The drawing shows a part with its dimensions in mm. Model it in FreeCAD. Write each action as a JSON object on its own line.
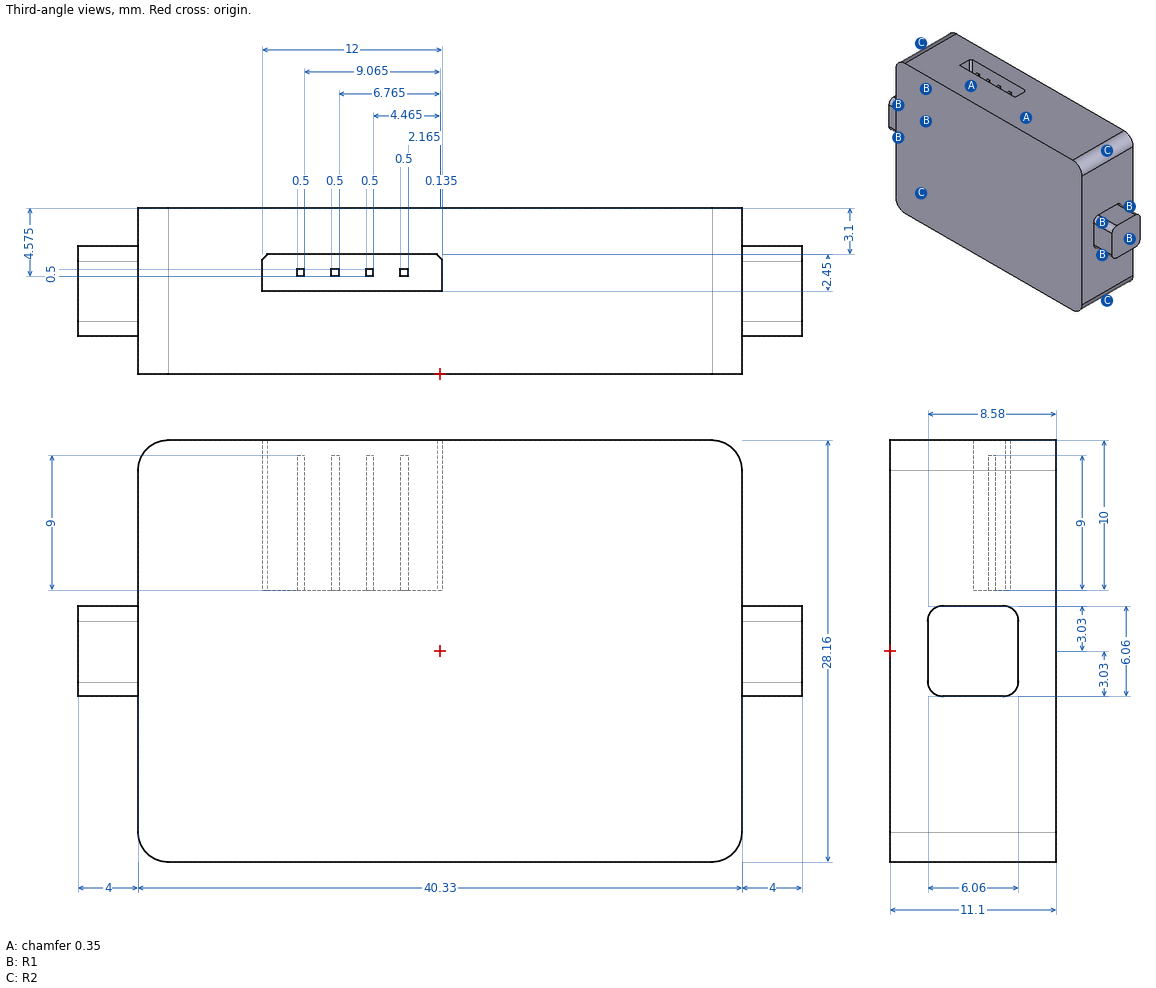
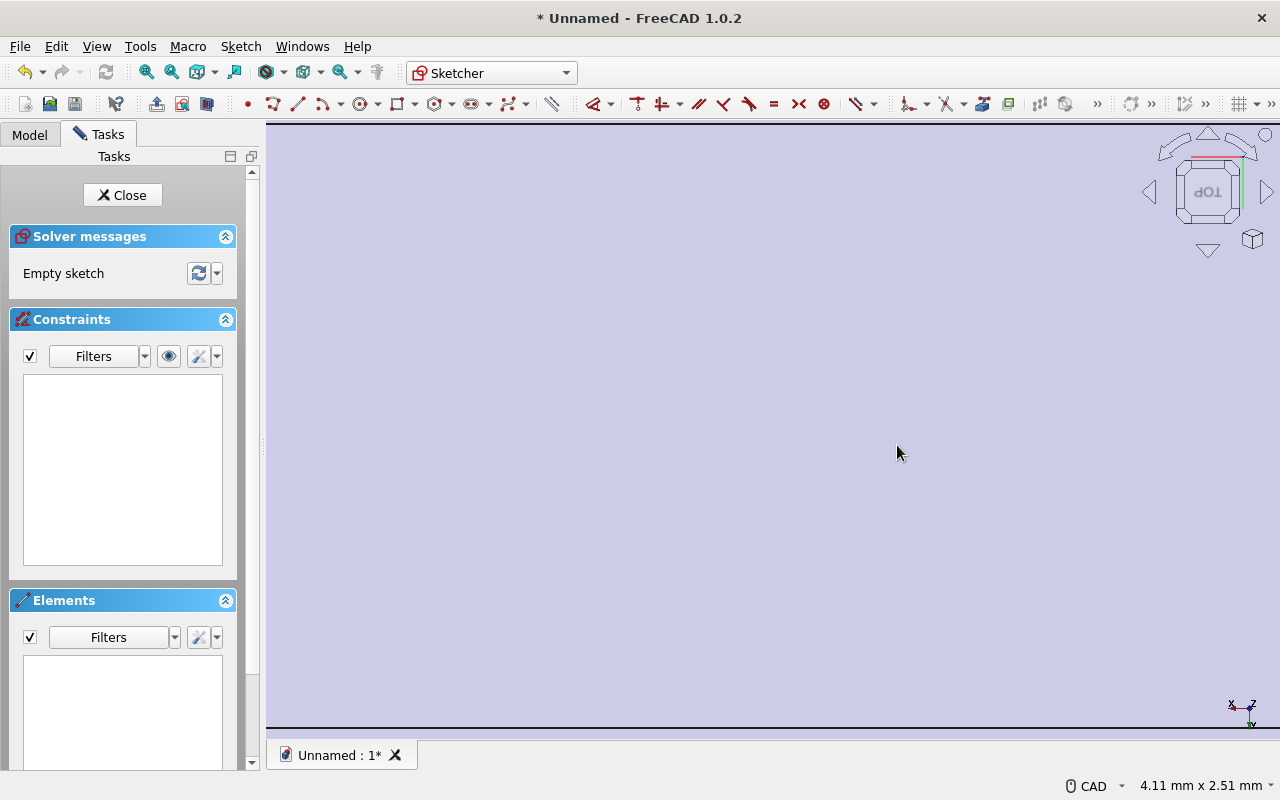
{"action": "scroll", "coordinate": [686, 424], "scroll_direction": "up", "scroll_amount": 6}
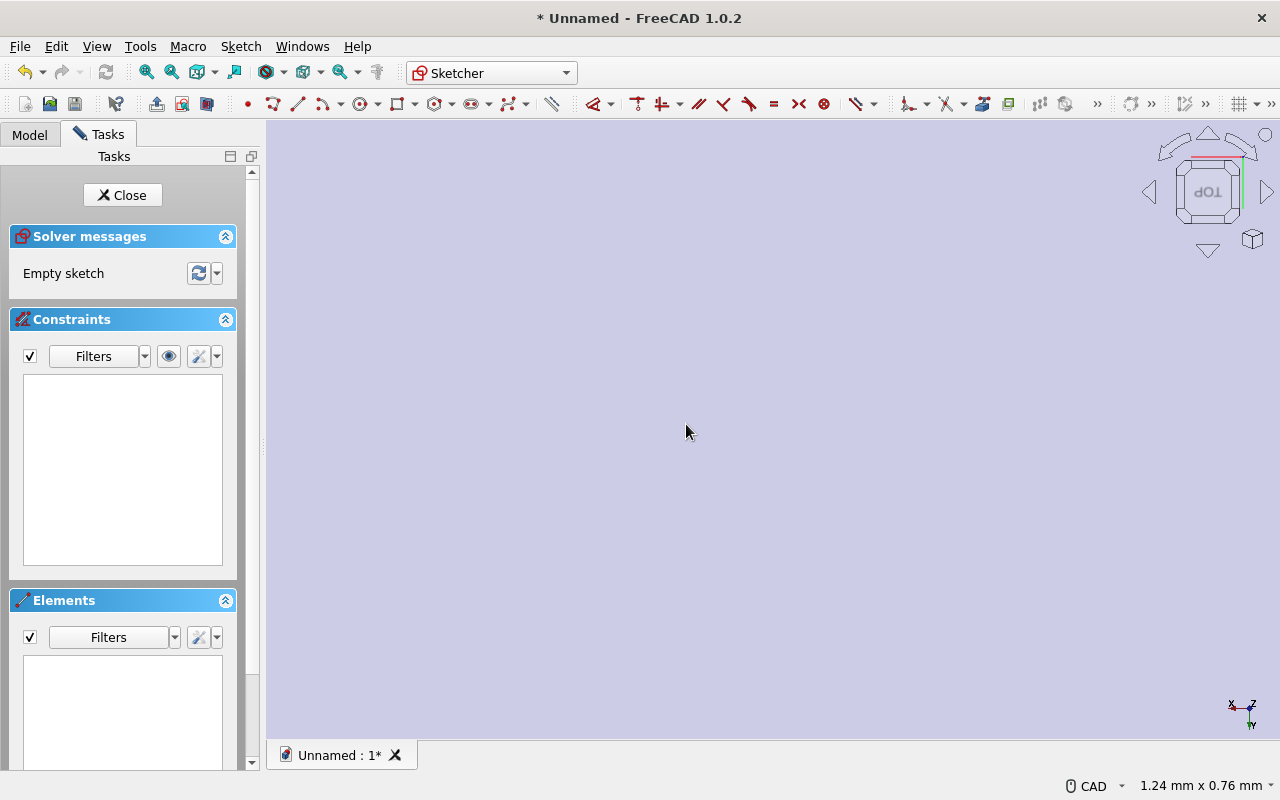
{"action": "left_click", "coordinate": [396, 104]}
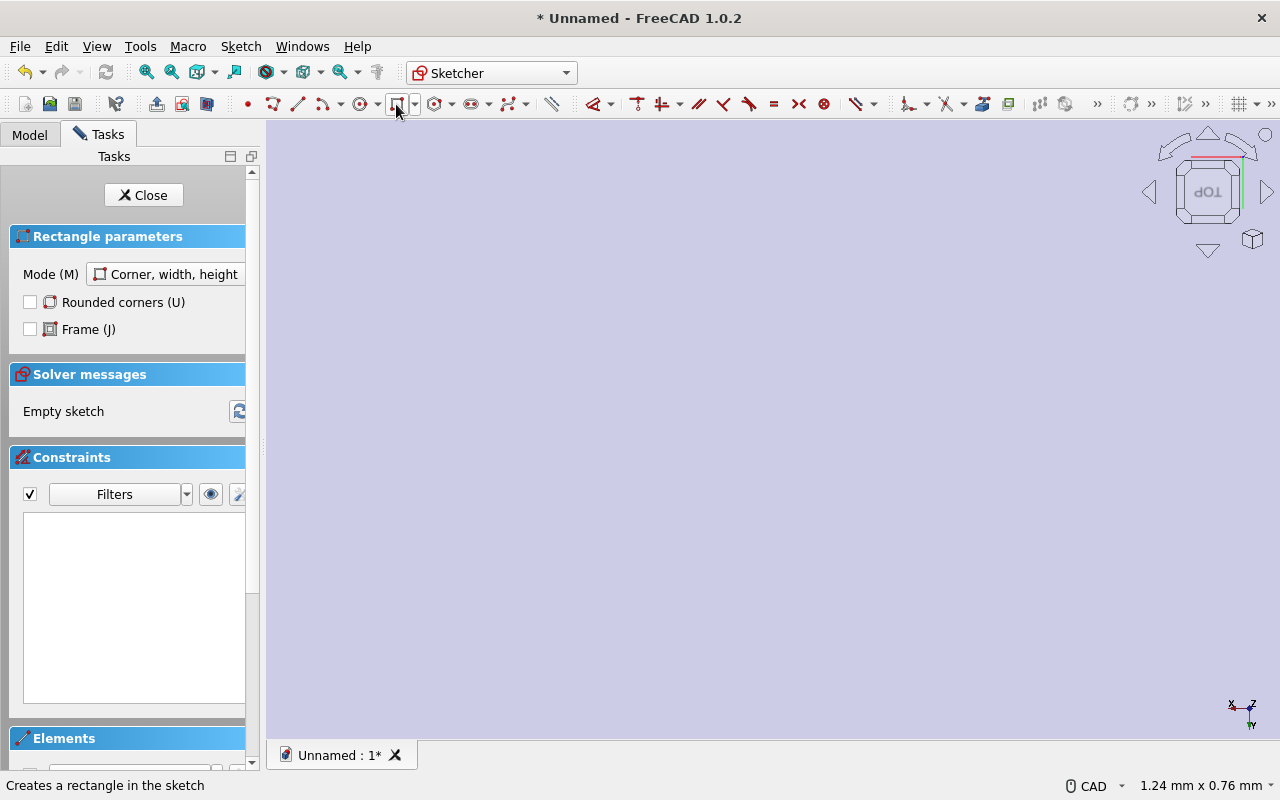
{"action": "left_click", "coordinate": [498, 224]}
{"action": "mouse_move", "coordinate": [907, 633]}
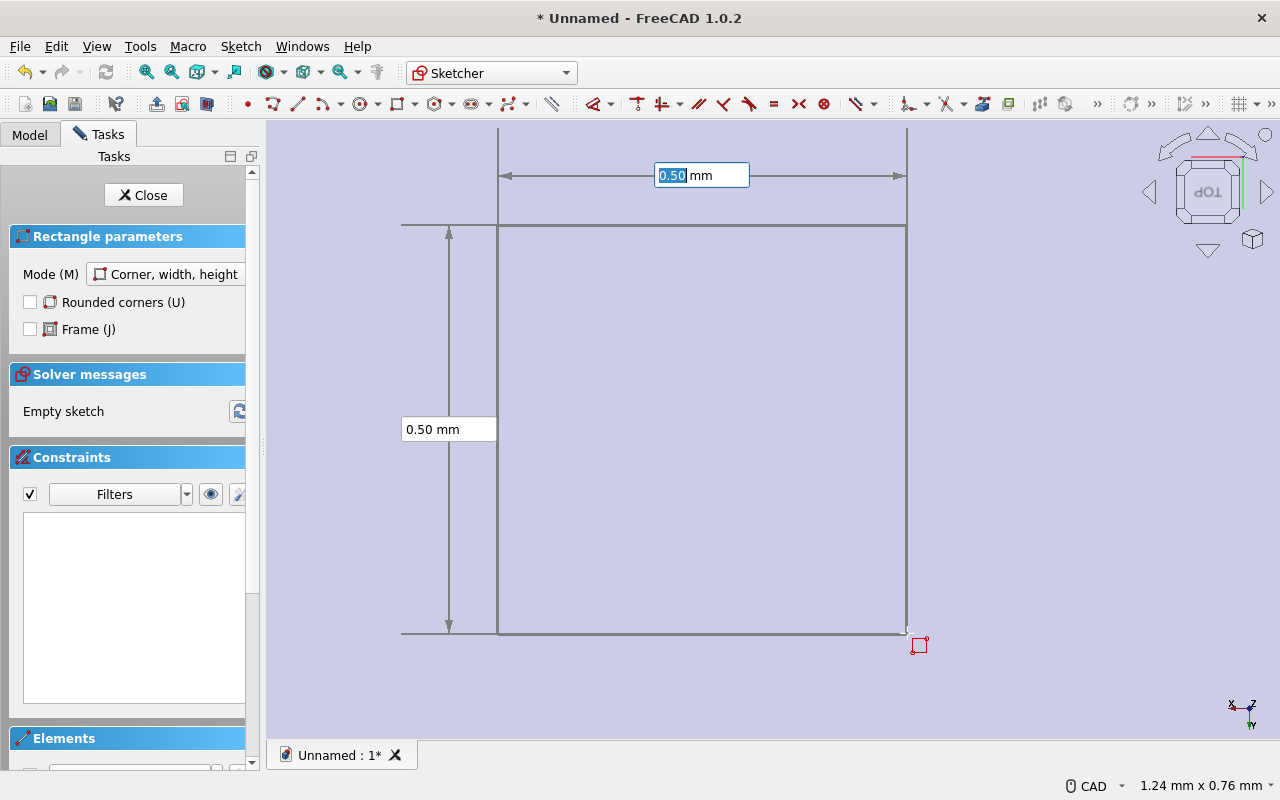
{"action": "type", "text": "0.5"}
{"action": "key", "text": "Tab"}
{"action": "type", "text": "0.5"}
{"action": "key", "text": "Return"}
{"action": "key", "text": "Escape"}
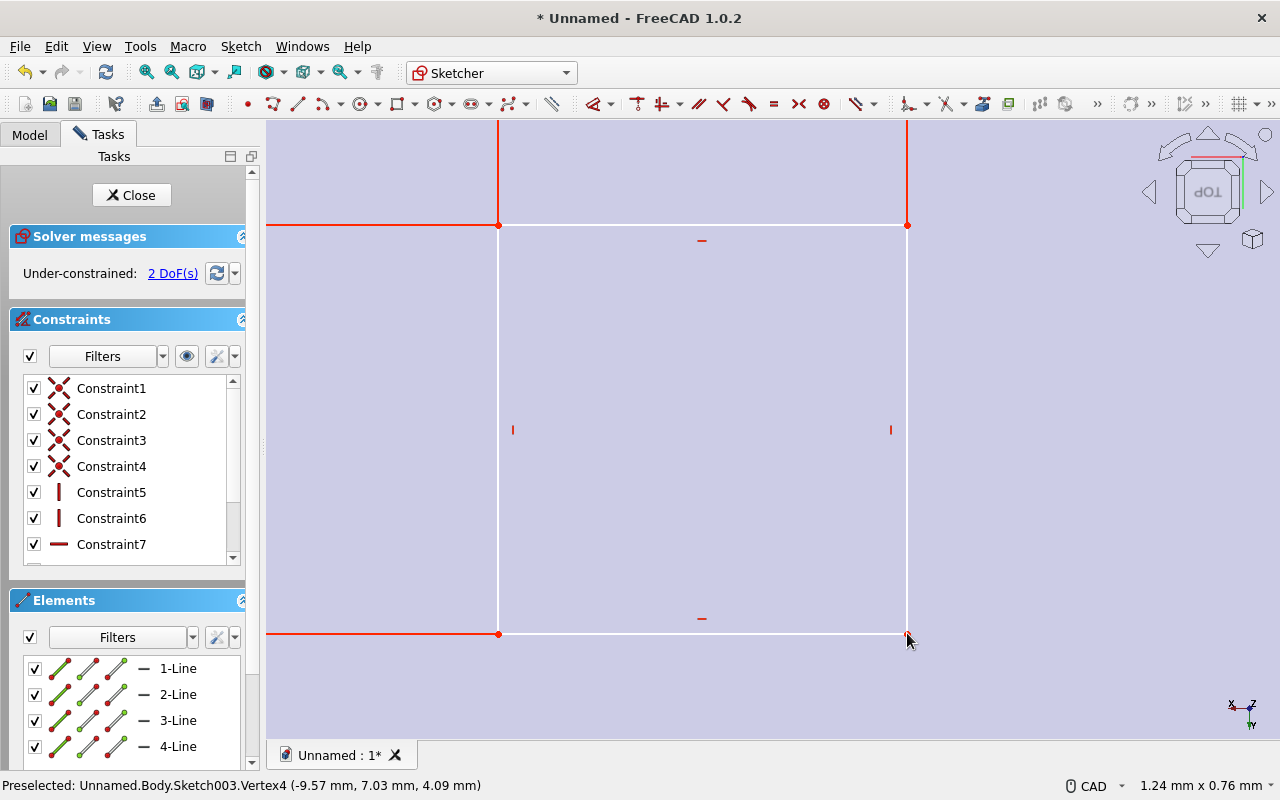
{"action": "left_click", "coordinate": [592, 104]}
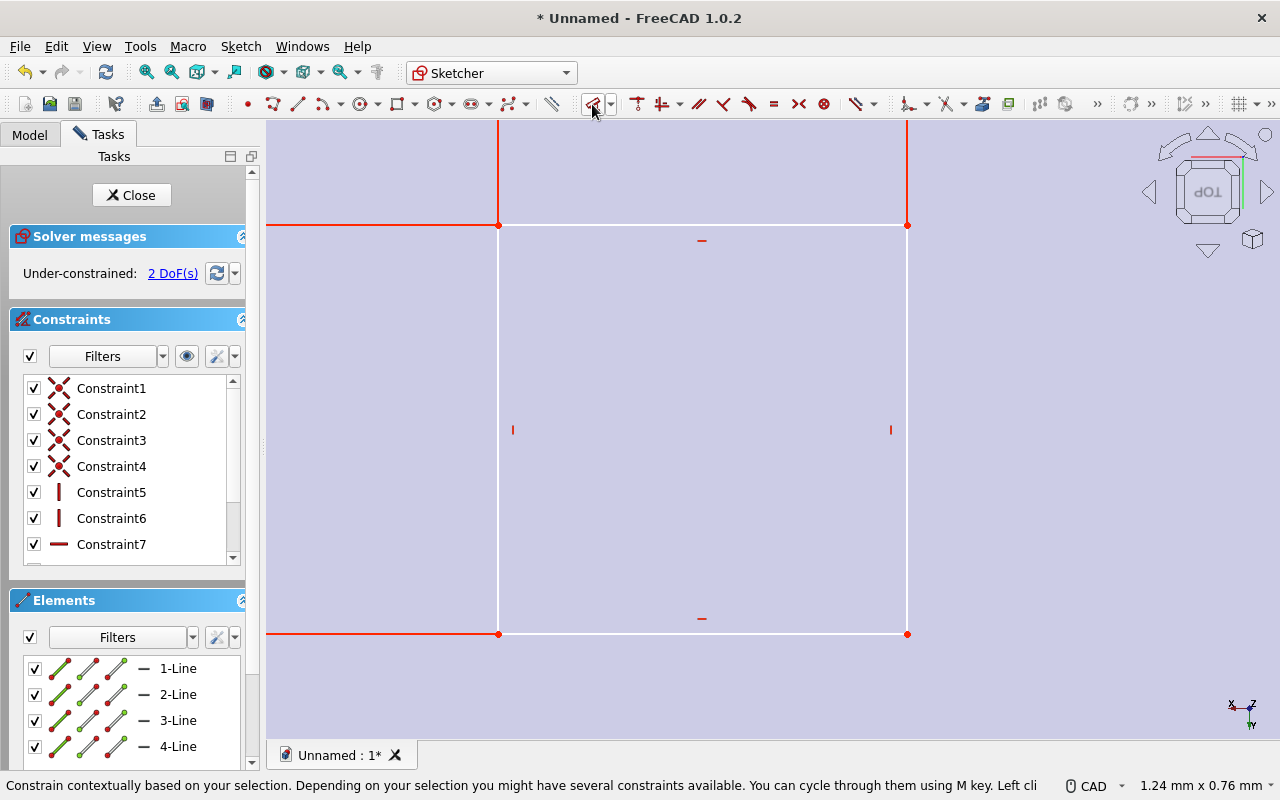
{"action": "left_click", "coordinate": [498, 225]}
{"action": "left_click", "coordinate": [396, 191]}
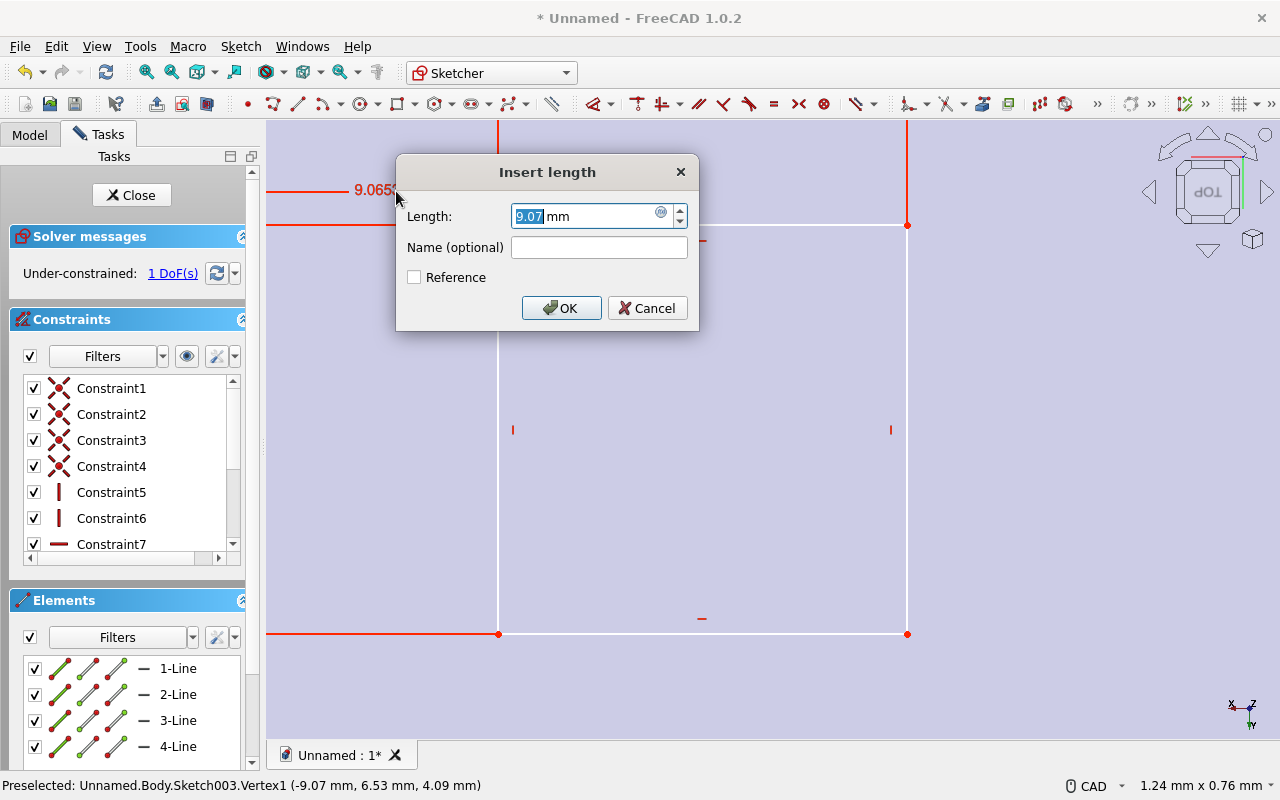
{"action": "type", "text": "9.065"}
{"action": "key", "text": "Return"}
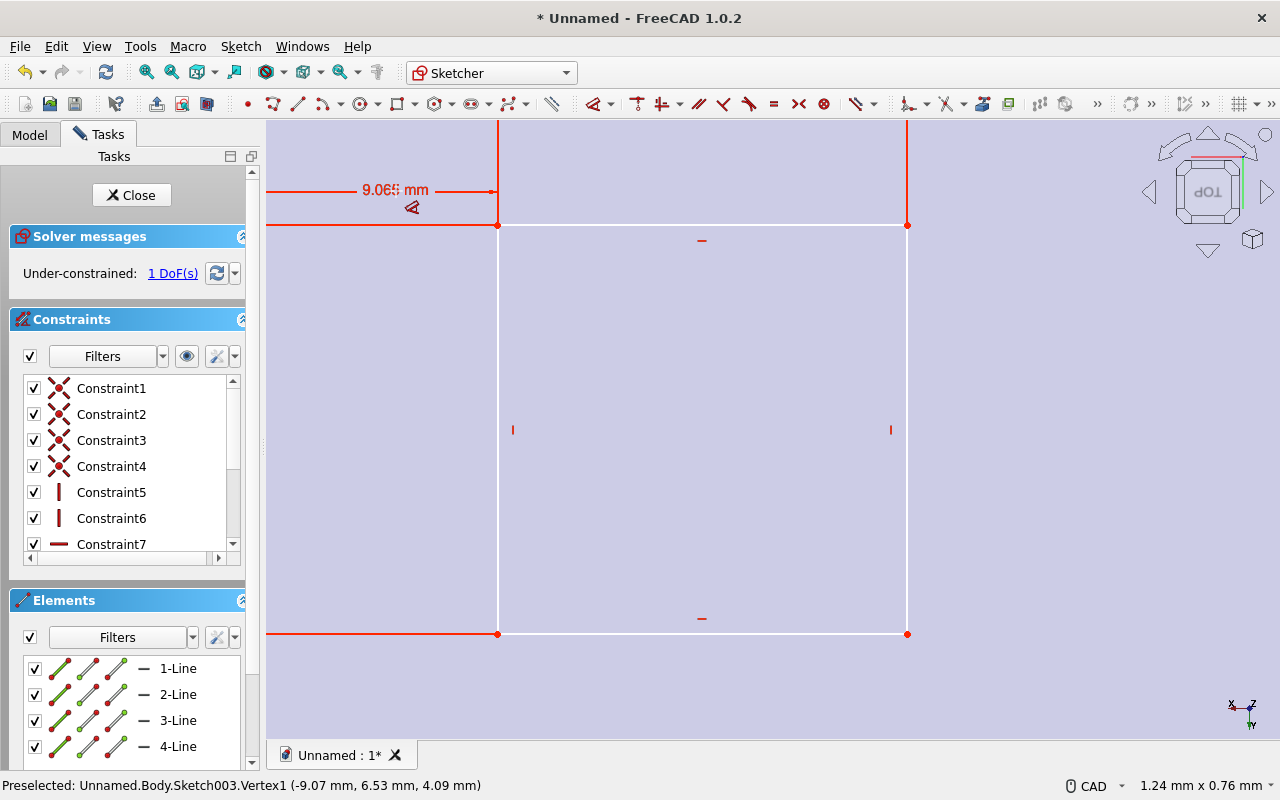
{"action": "left_click", "coordinate": [498, 225]}
{"action": "left_click", "coordinate": [532, 468]}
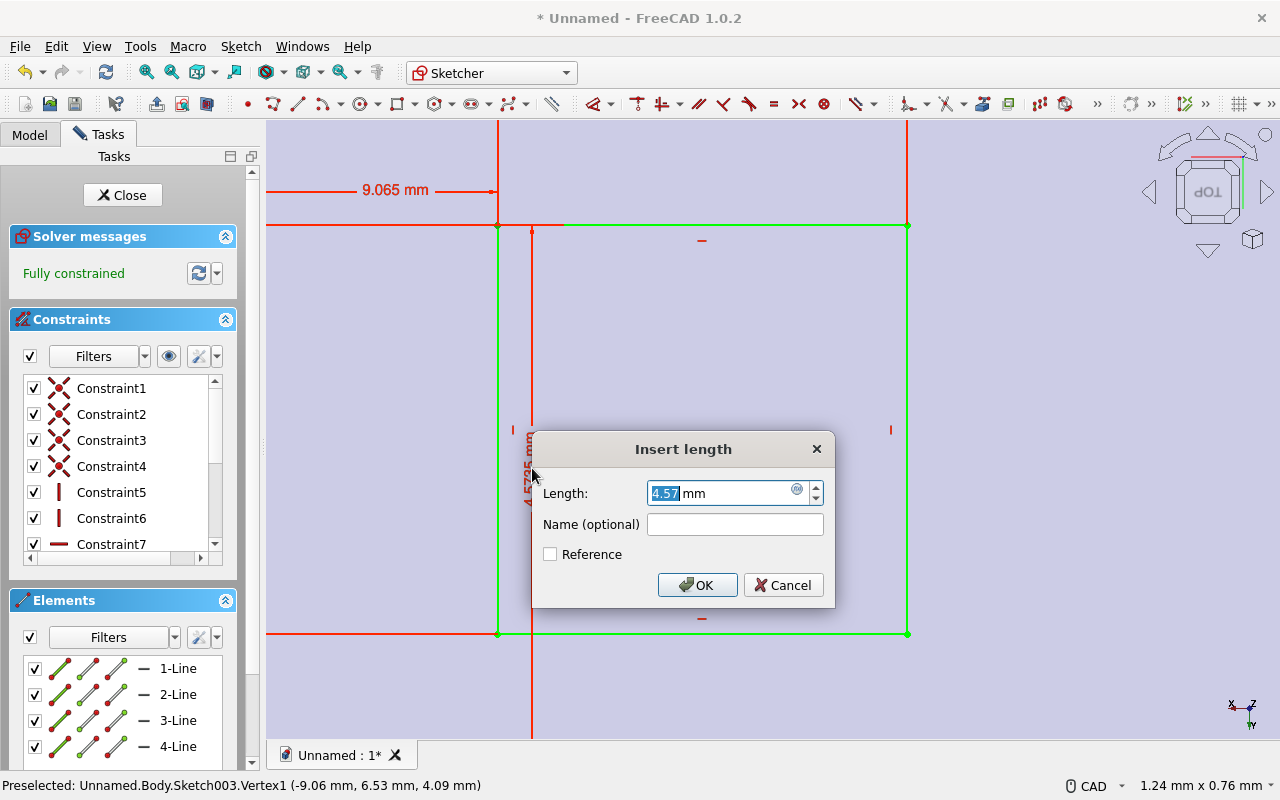
{"action": "type", "text": "4.575"}
{"action": "key", "text": "Return"}
{"action": "key", "text": "Escape"}